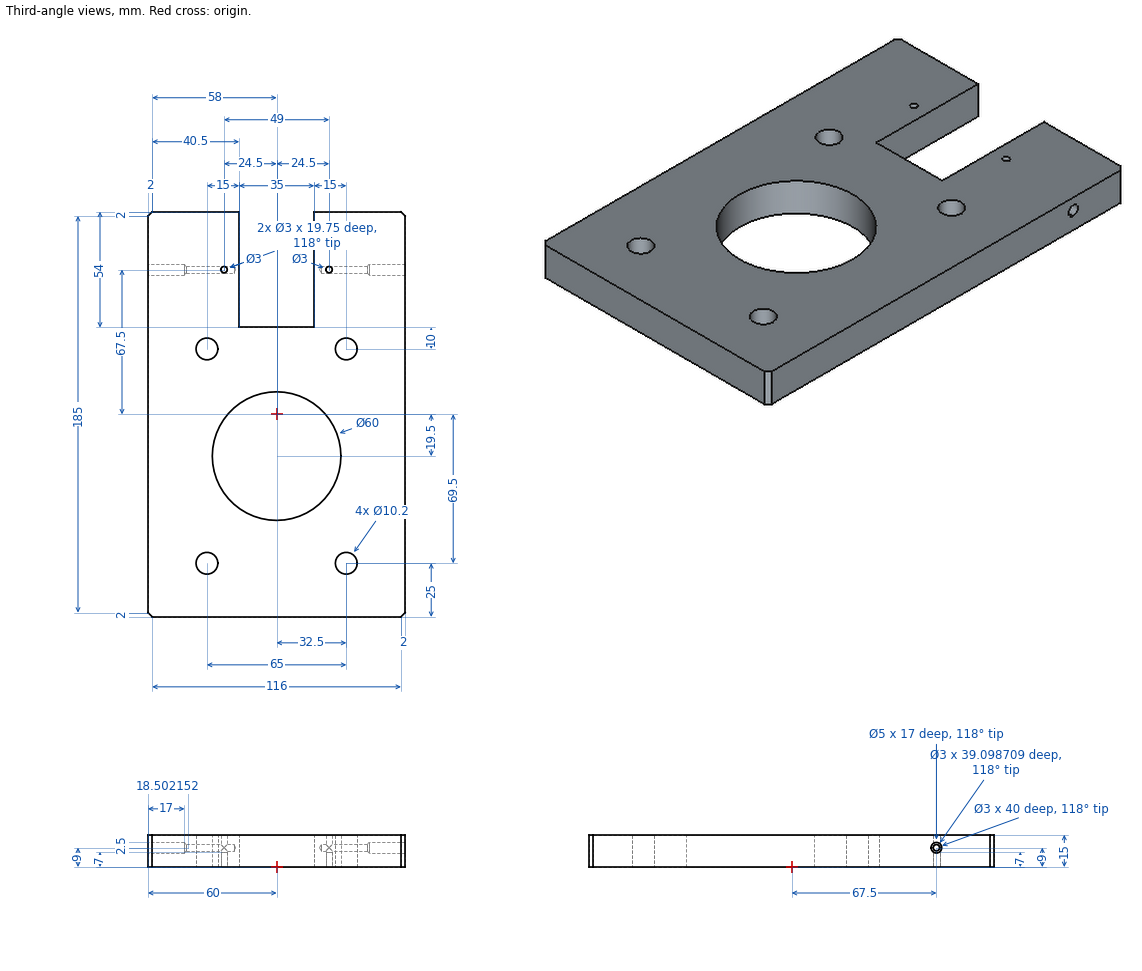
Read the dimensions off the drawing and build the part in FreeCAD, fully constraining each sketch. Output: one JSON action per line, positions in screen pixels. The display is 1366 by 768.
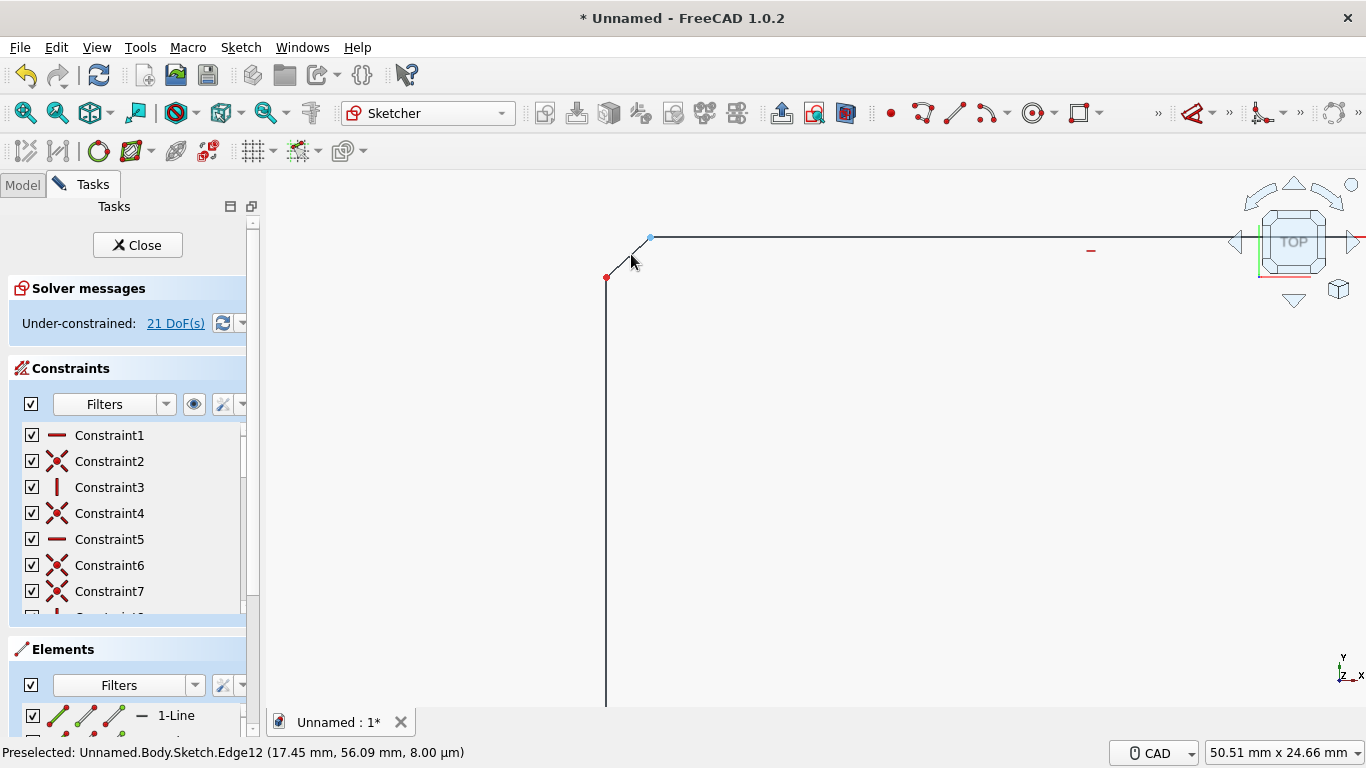
{"action": "left_click", "coordinate": [629, 257]}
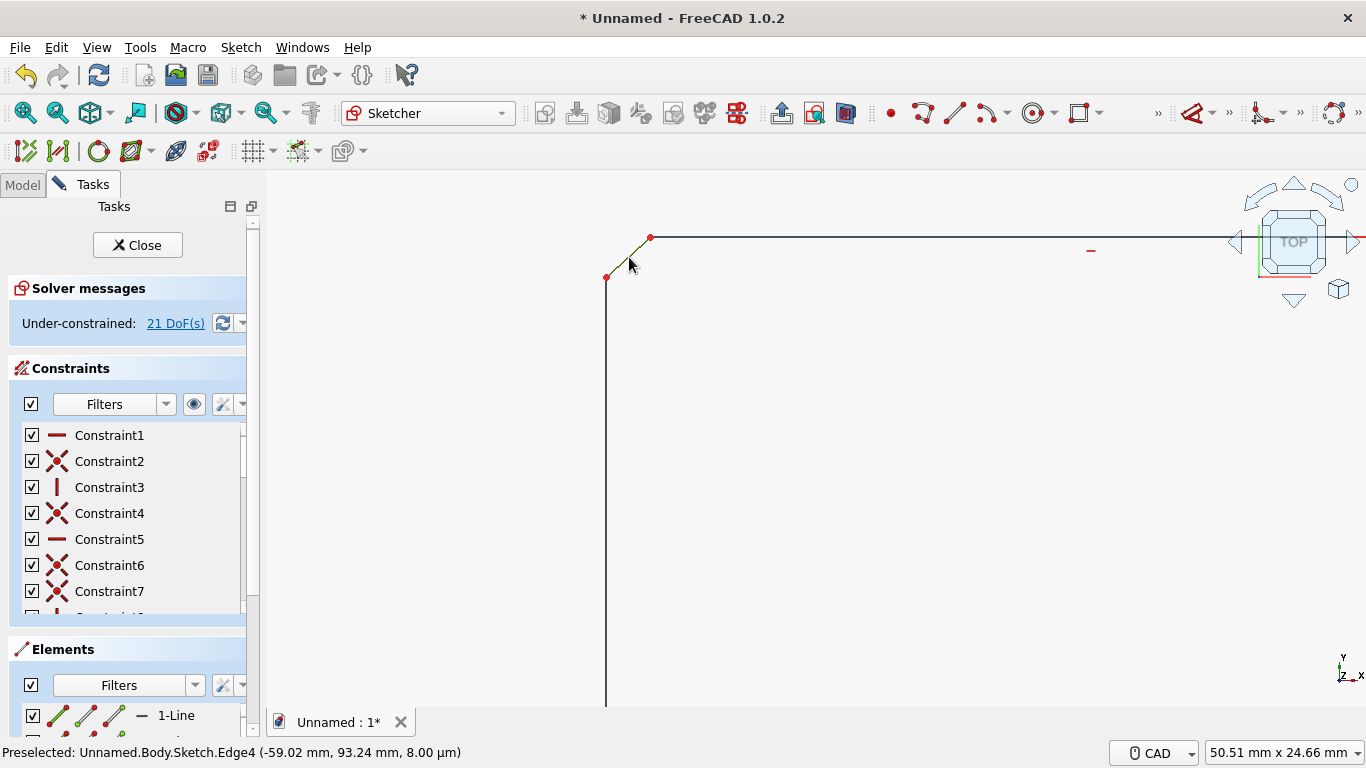
{"action": "left_click", "coordinate": [1214, 114]}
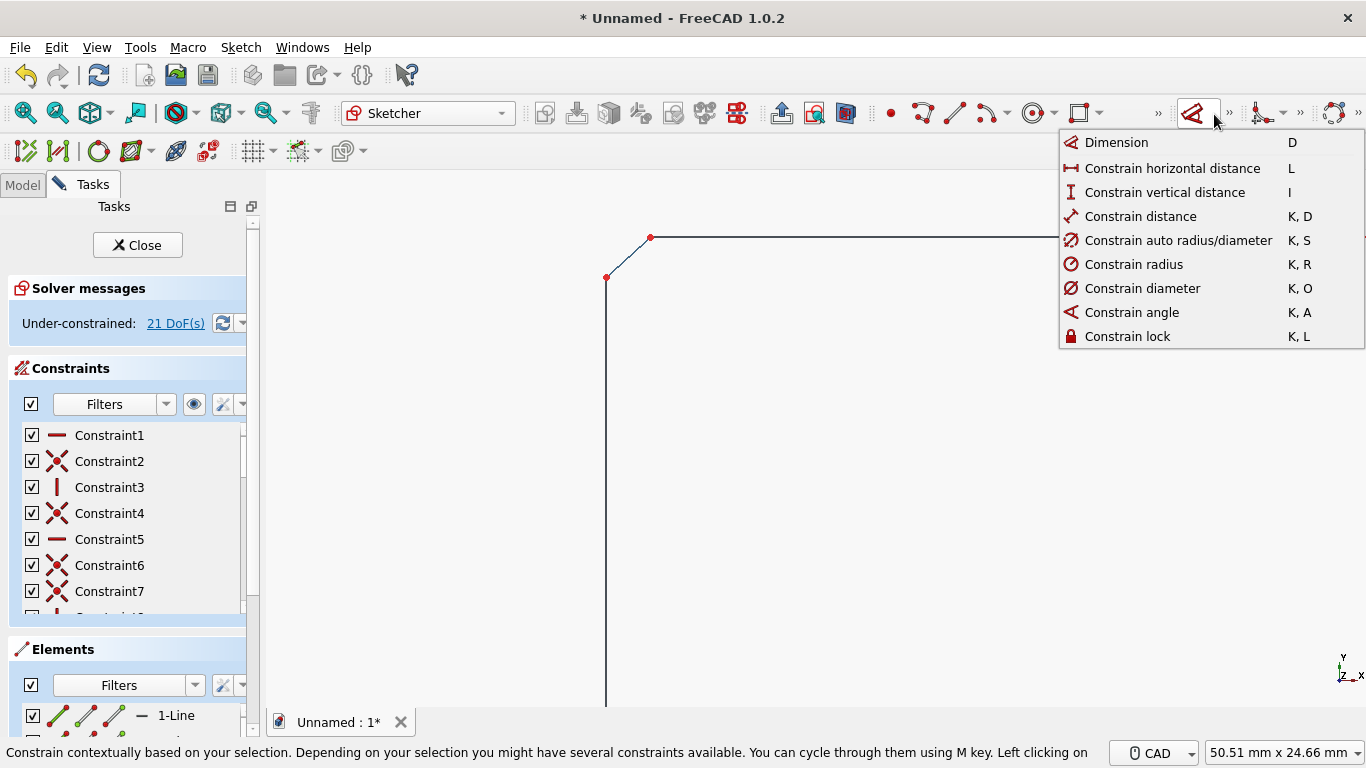
{"action": "left_click", "coordinate": [1212, 168]}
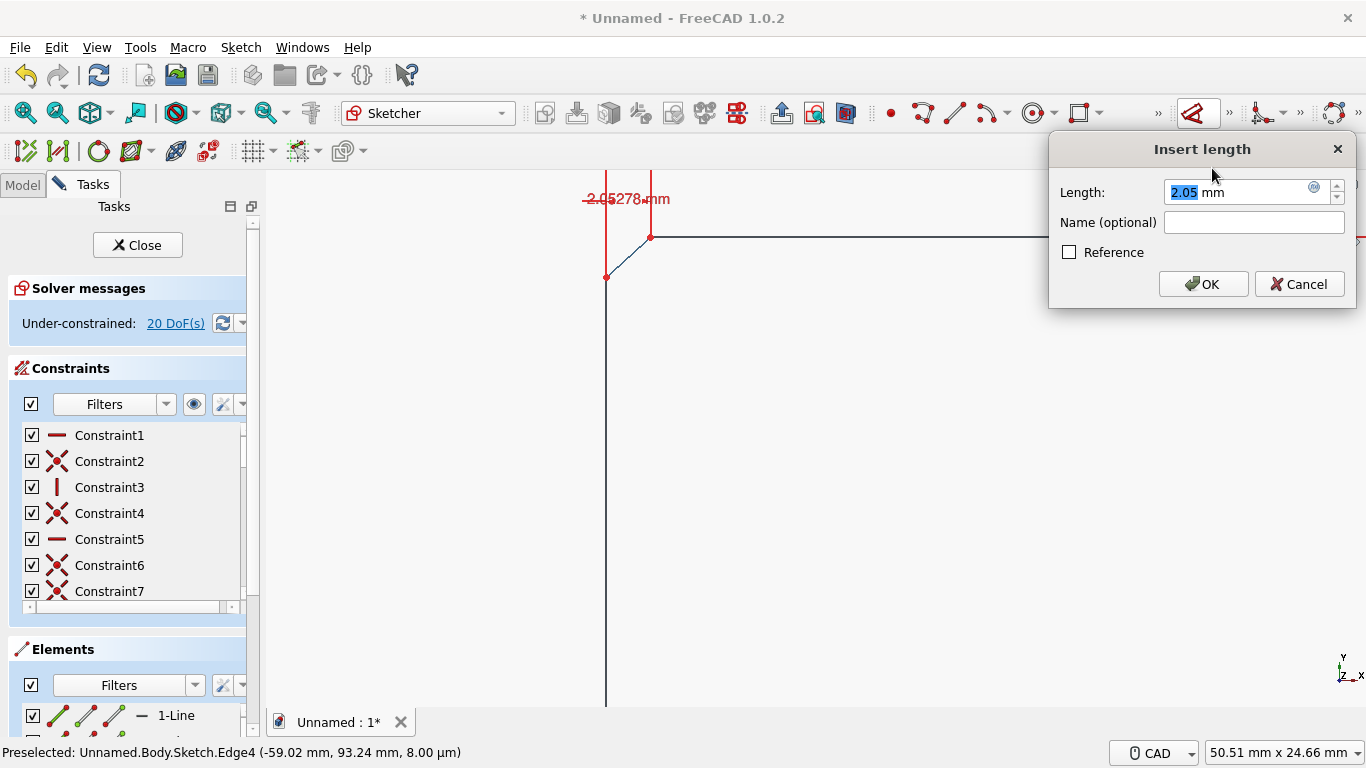
{"action": "type", "text": "2"}
{"action": "key", "text": "Return"}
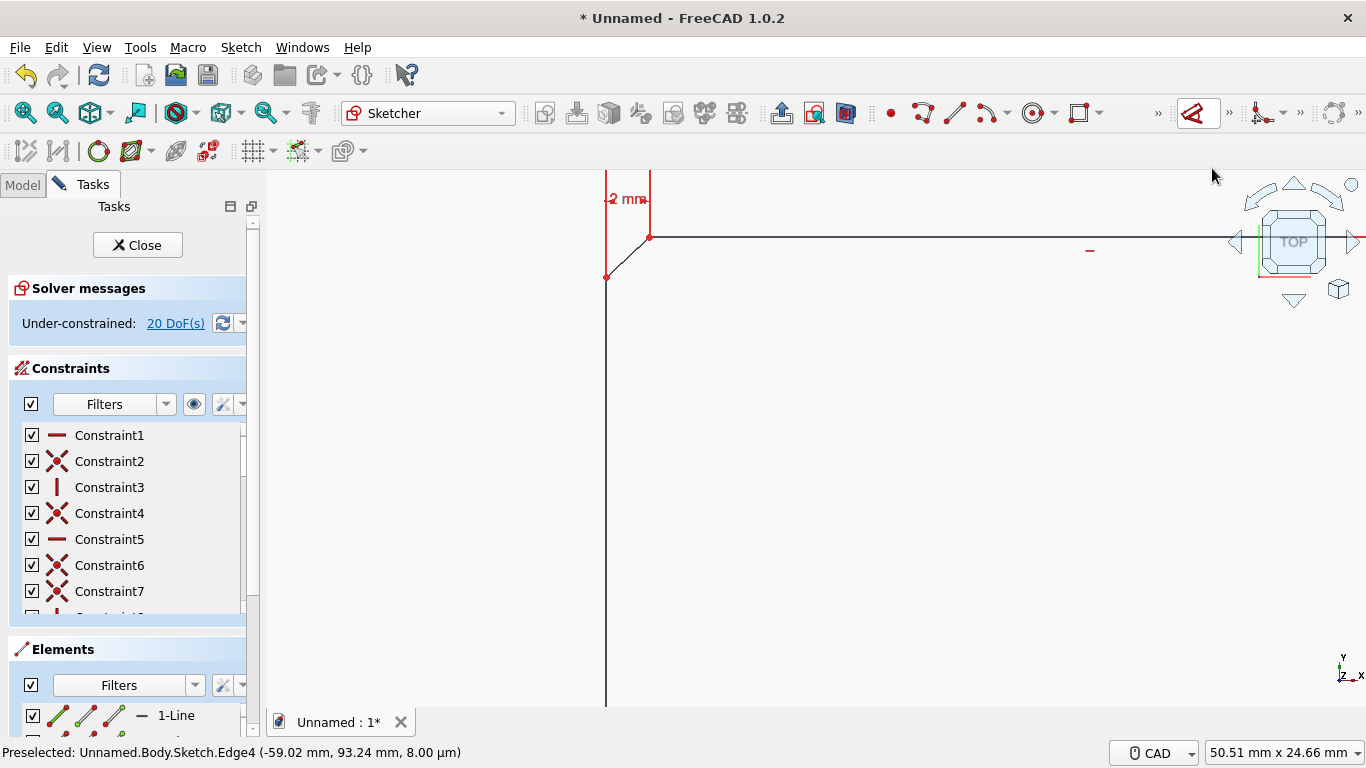
{"action": "left_click", "coordinate": [637, 249]}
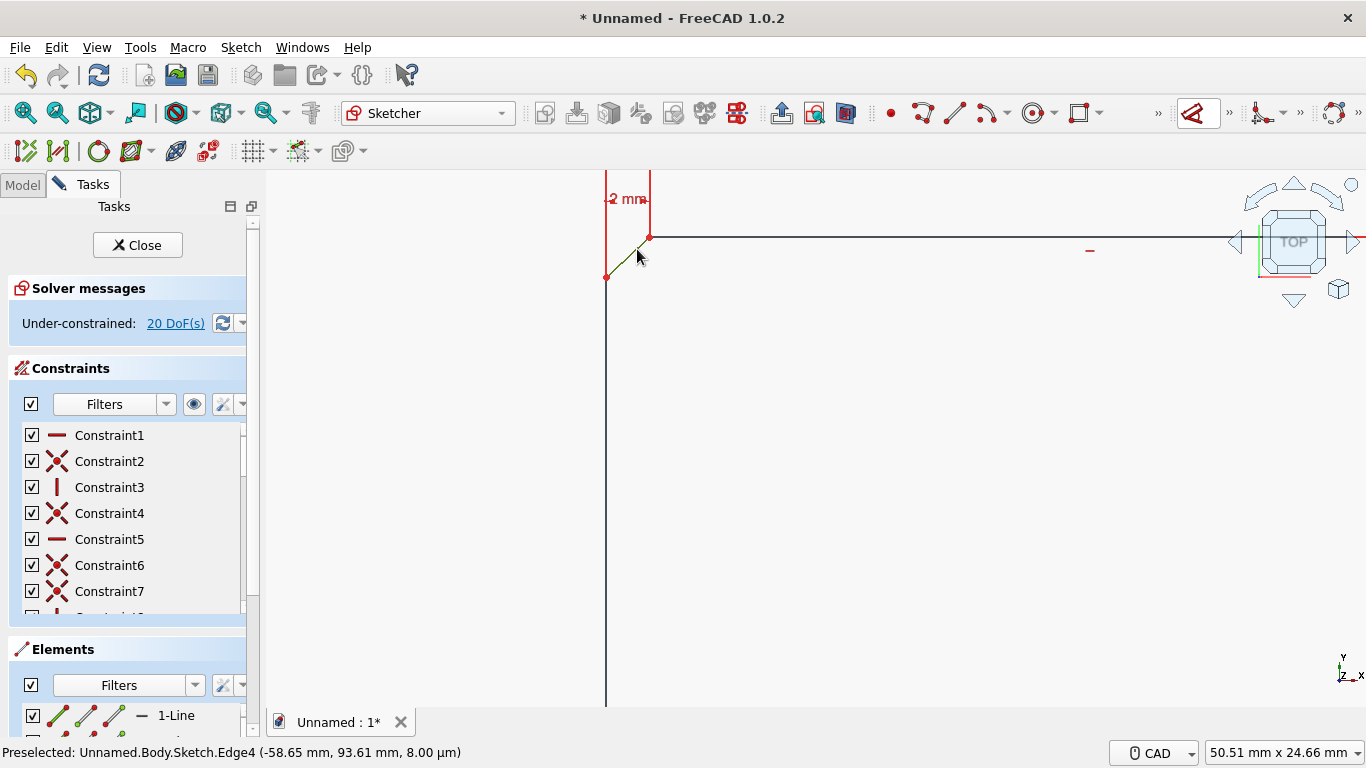
{"action": "key", "text": "i"}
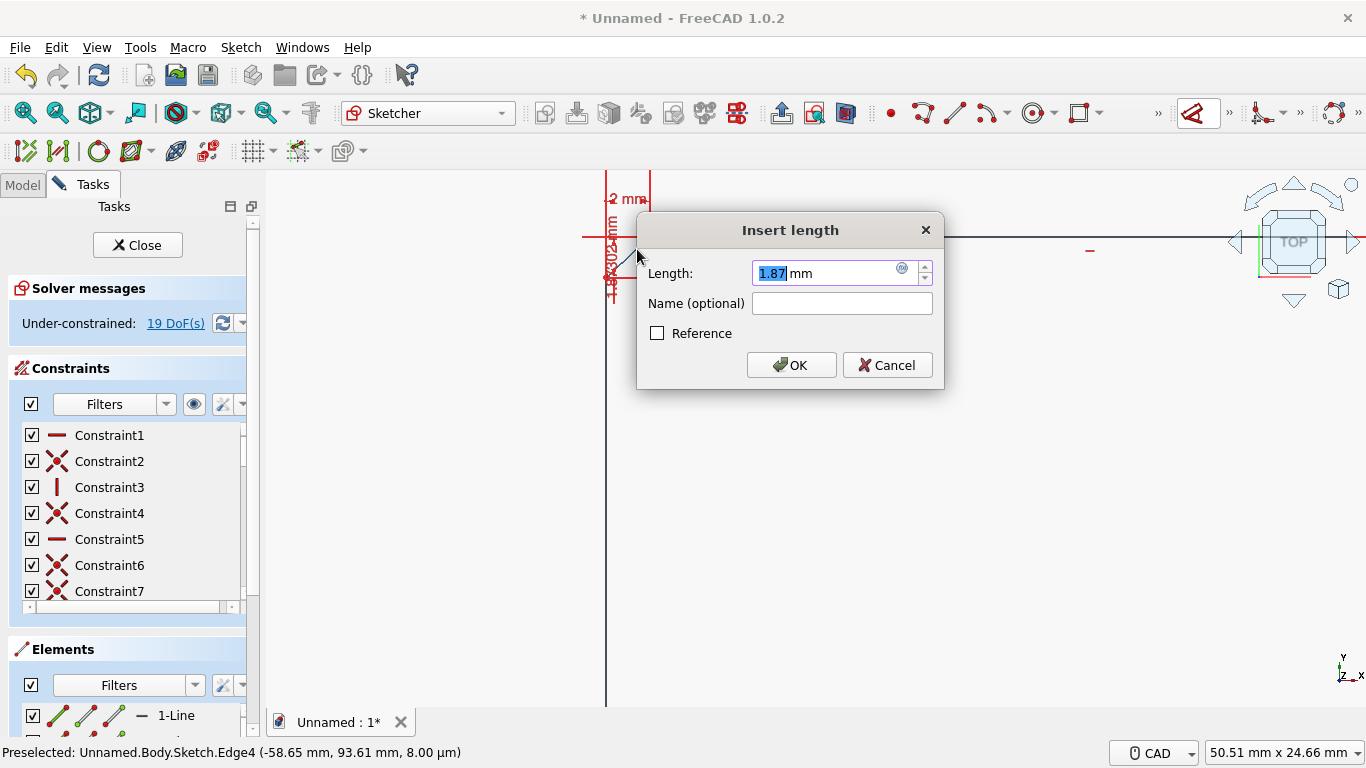
{"action": "type", "text": "2"}
{"action": "key", "text": "Return"}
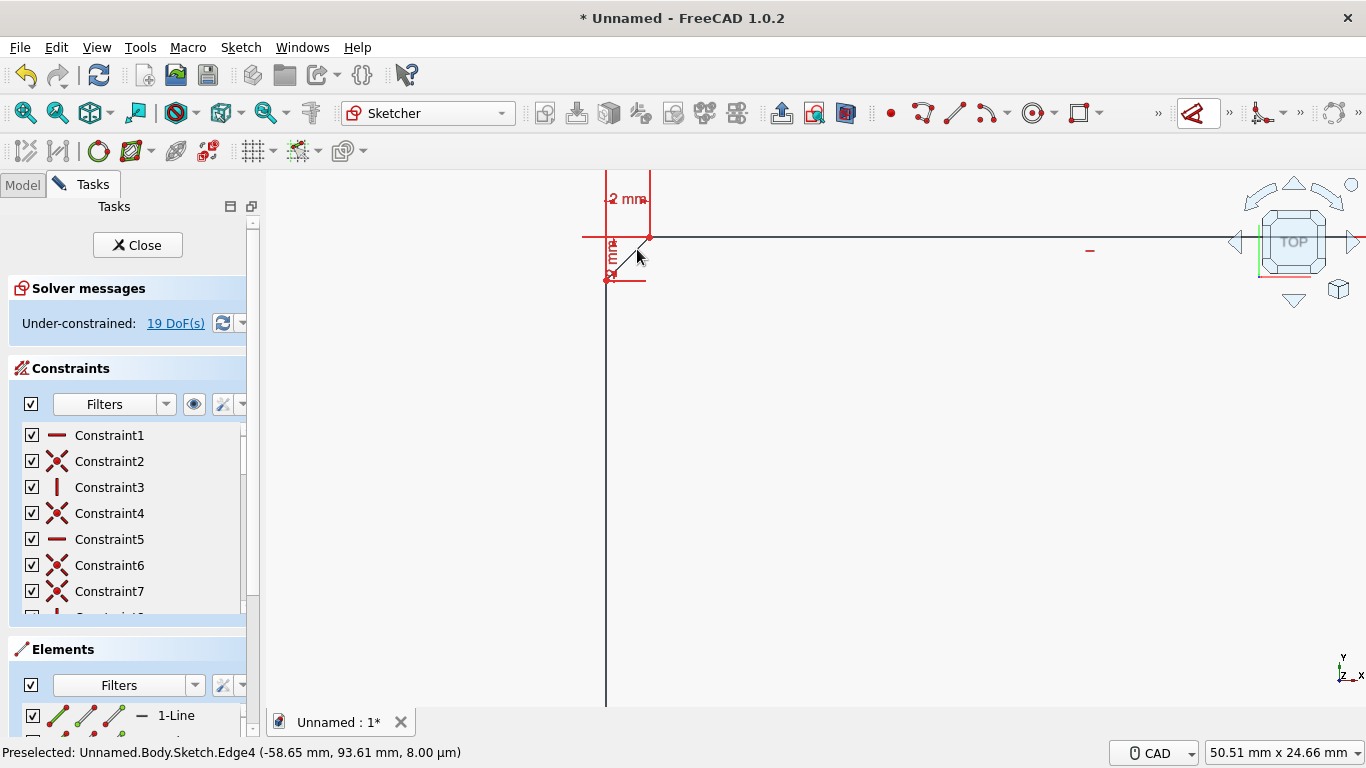
{"action": "scroll", "coordinate": [631, 254], "scroll_direction": "down", "scroll_amount": 12}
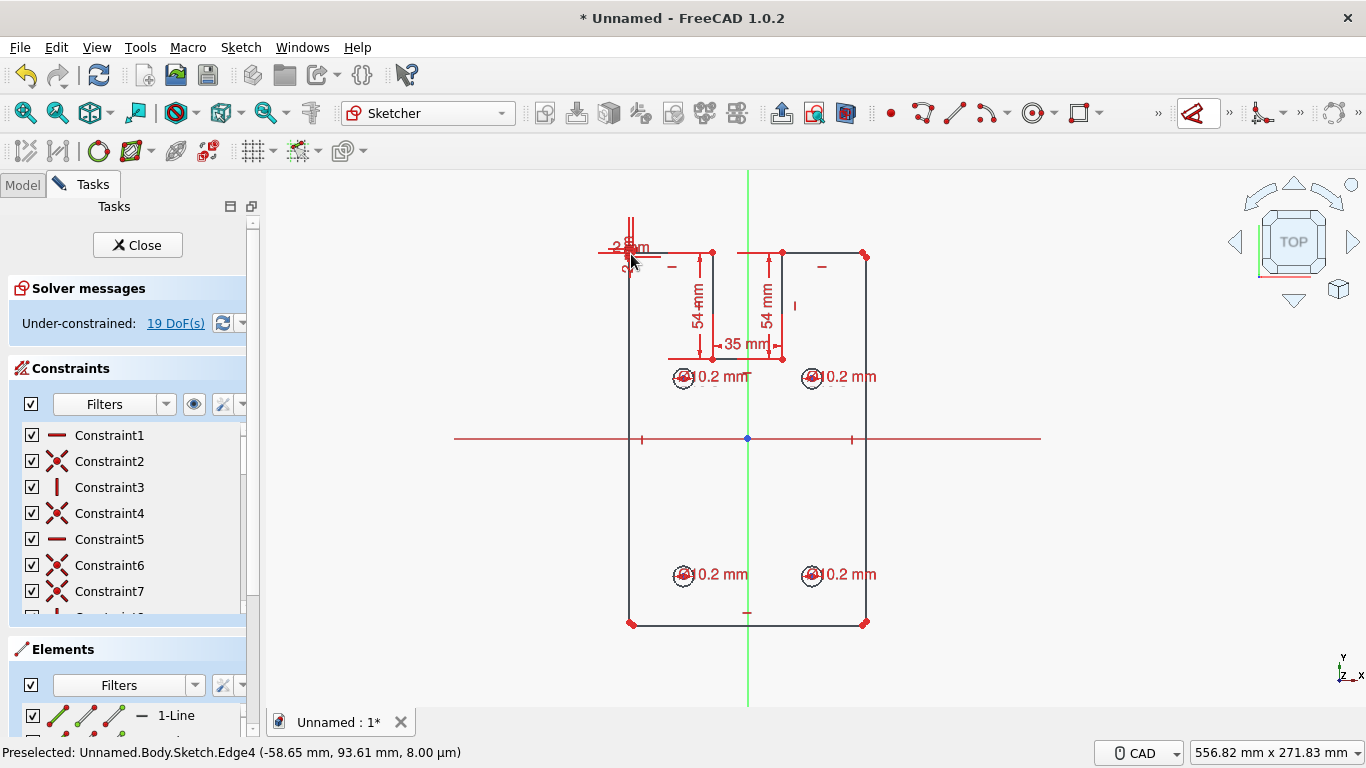
{"action": "scroll", "coordinate": [630, 623], "scroll_direction": "up", "scroll_amount": 12}